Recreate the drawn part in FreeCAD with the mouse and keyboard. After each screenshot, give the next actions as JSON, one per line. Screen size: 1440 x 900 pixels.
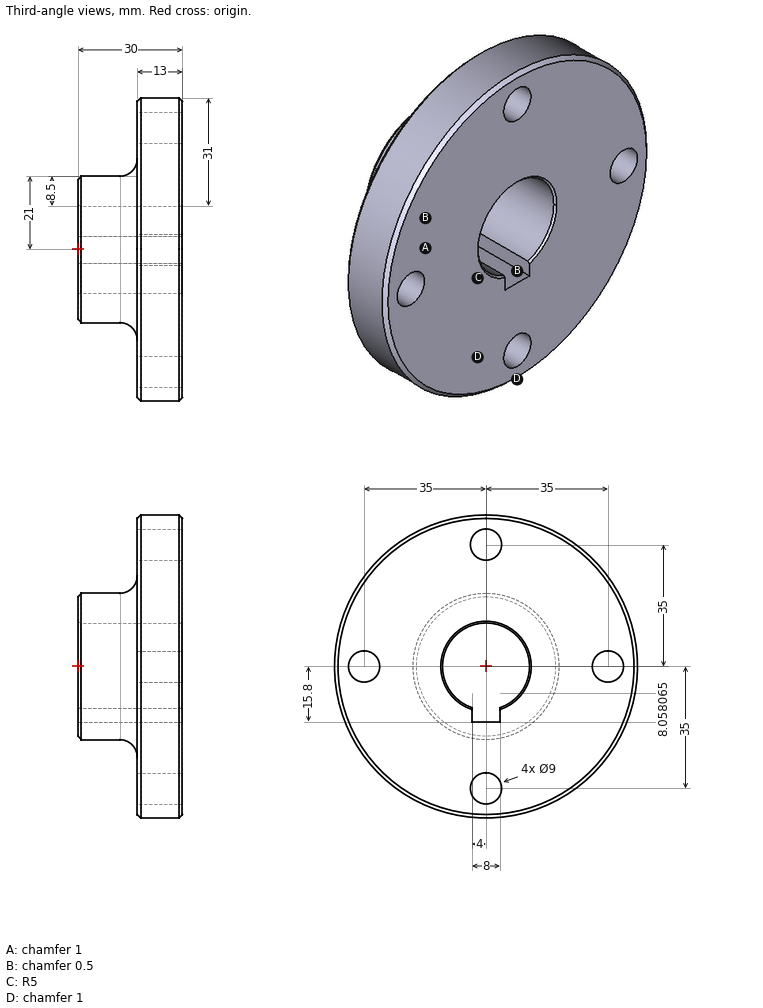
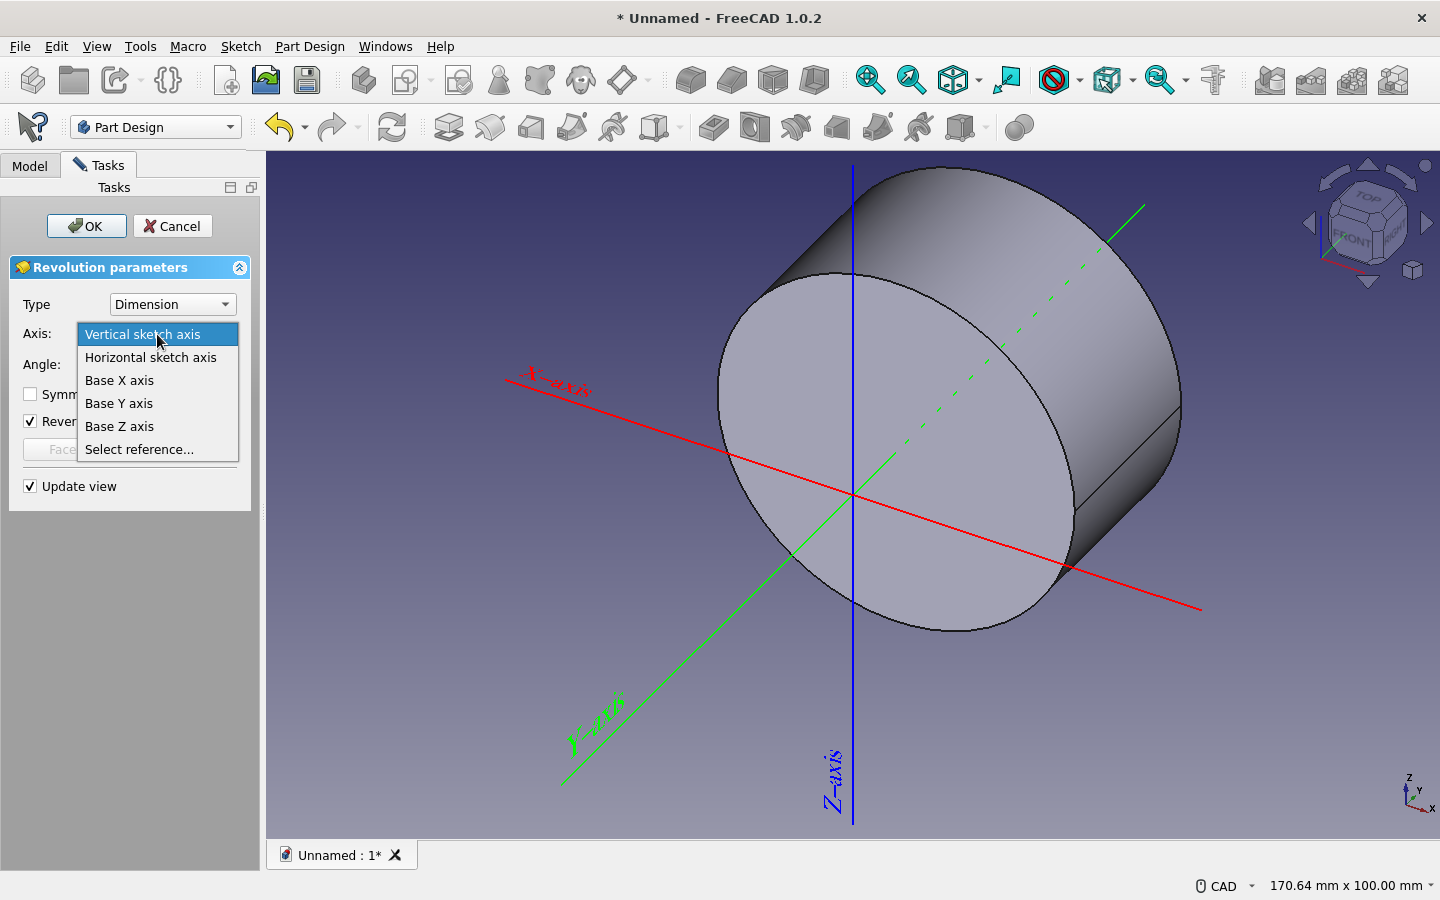
{"action": "left_click", "coordinate": [156, 358]}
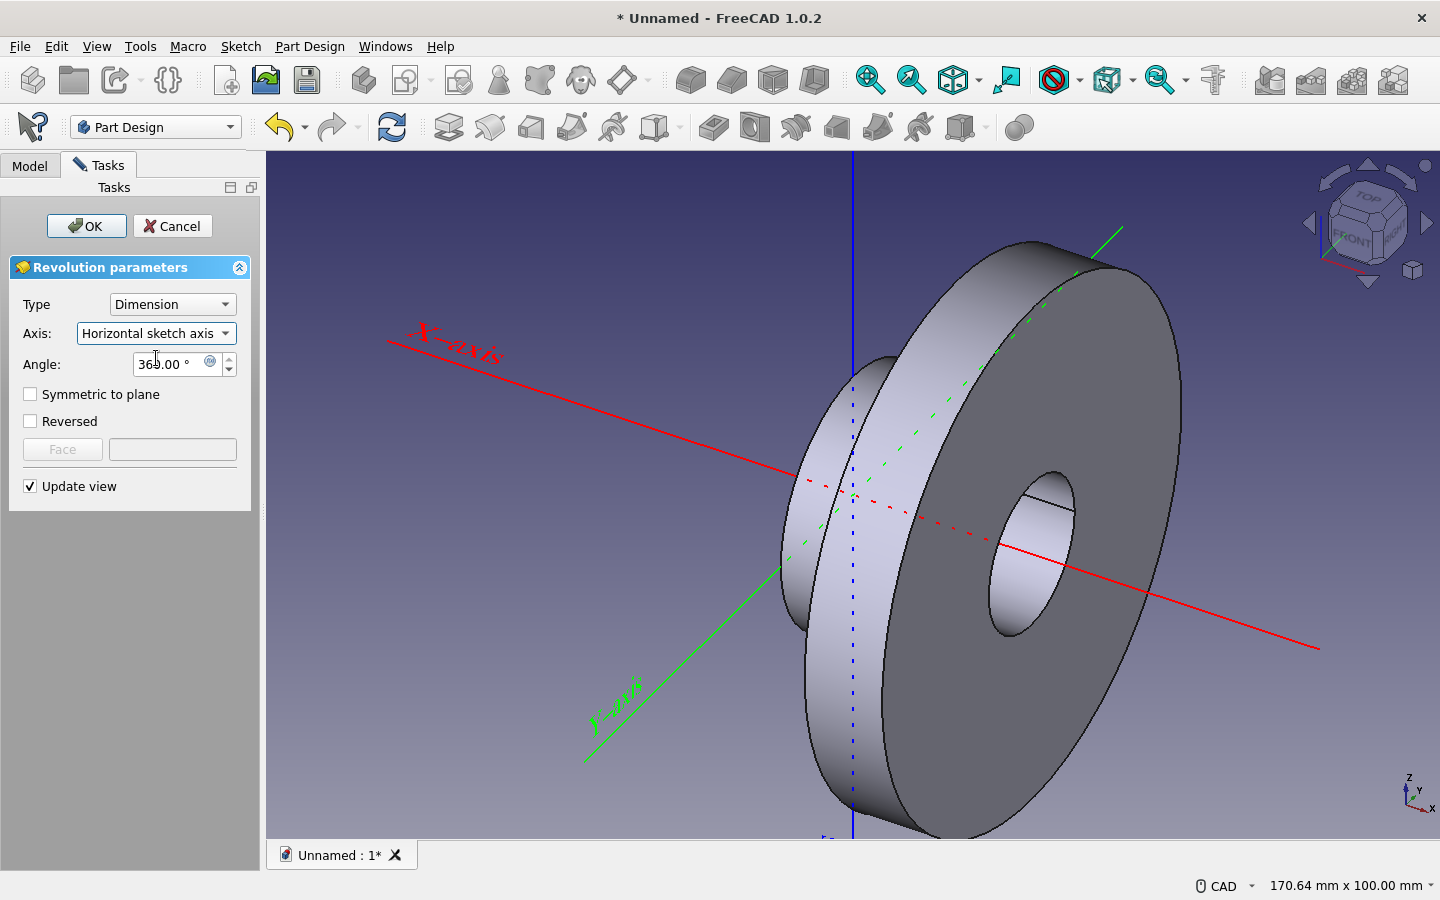
{"action": "left_click", "coordinate": [87, 226]}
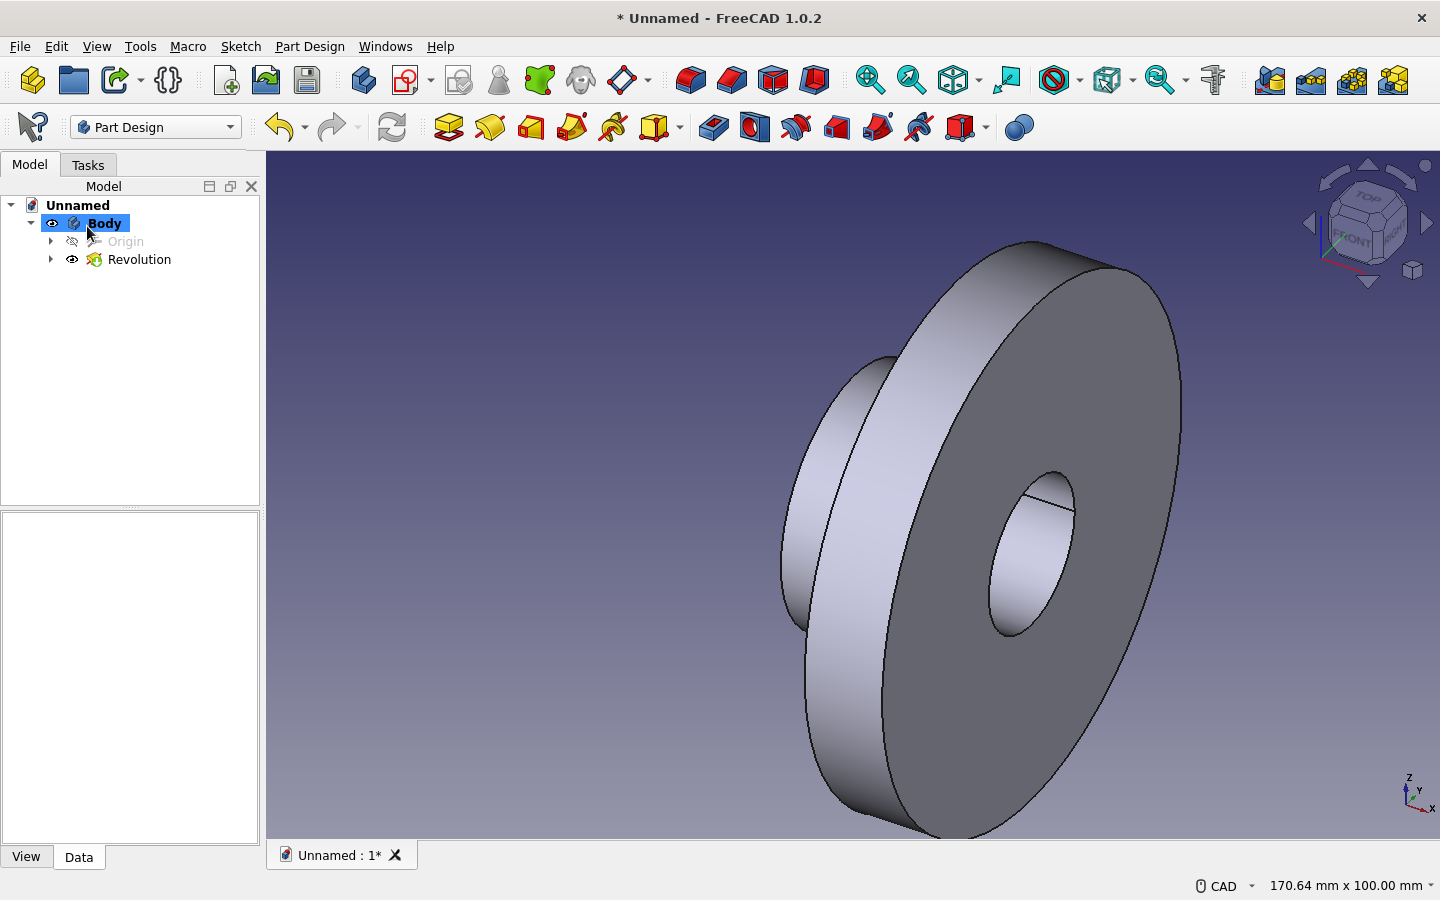
{"action": "left_click", "coordinate": [871, 80]}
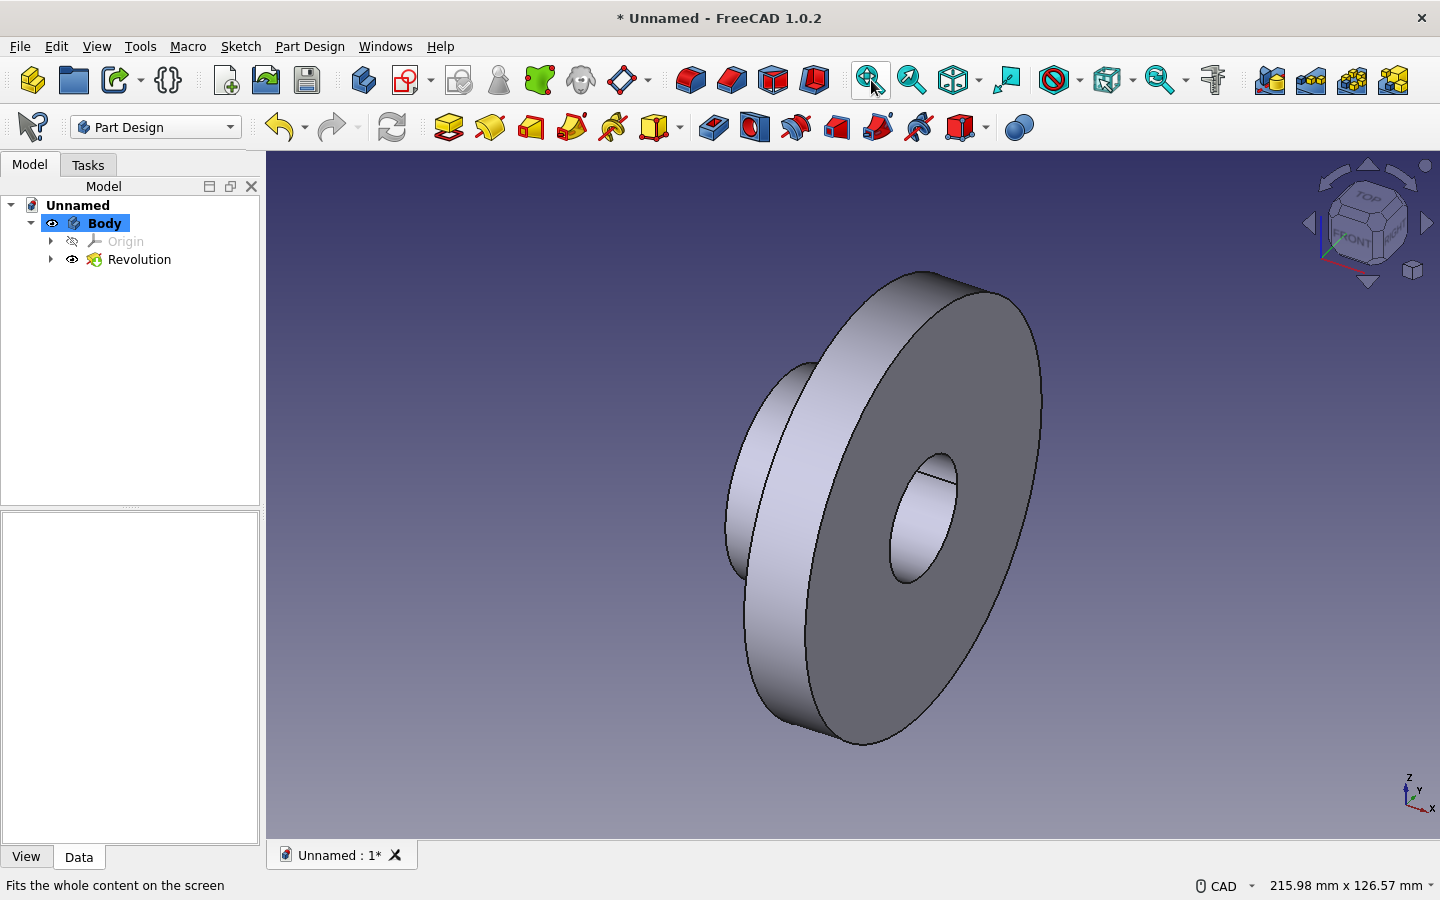
{"action": "key", "text": "0"}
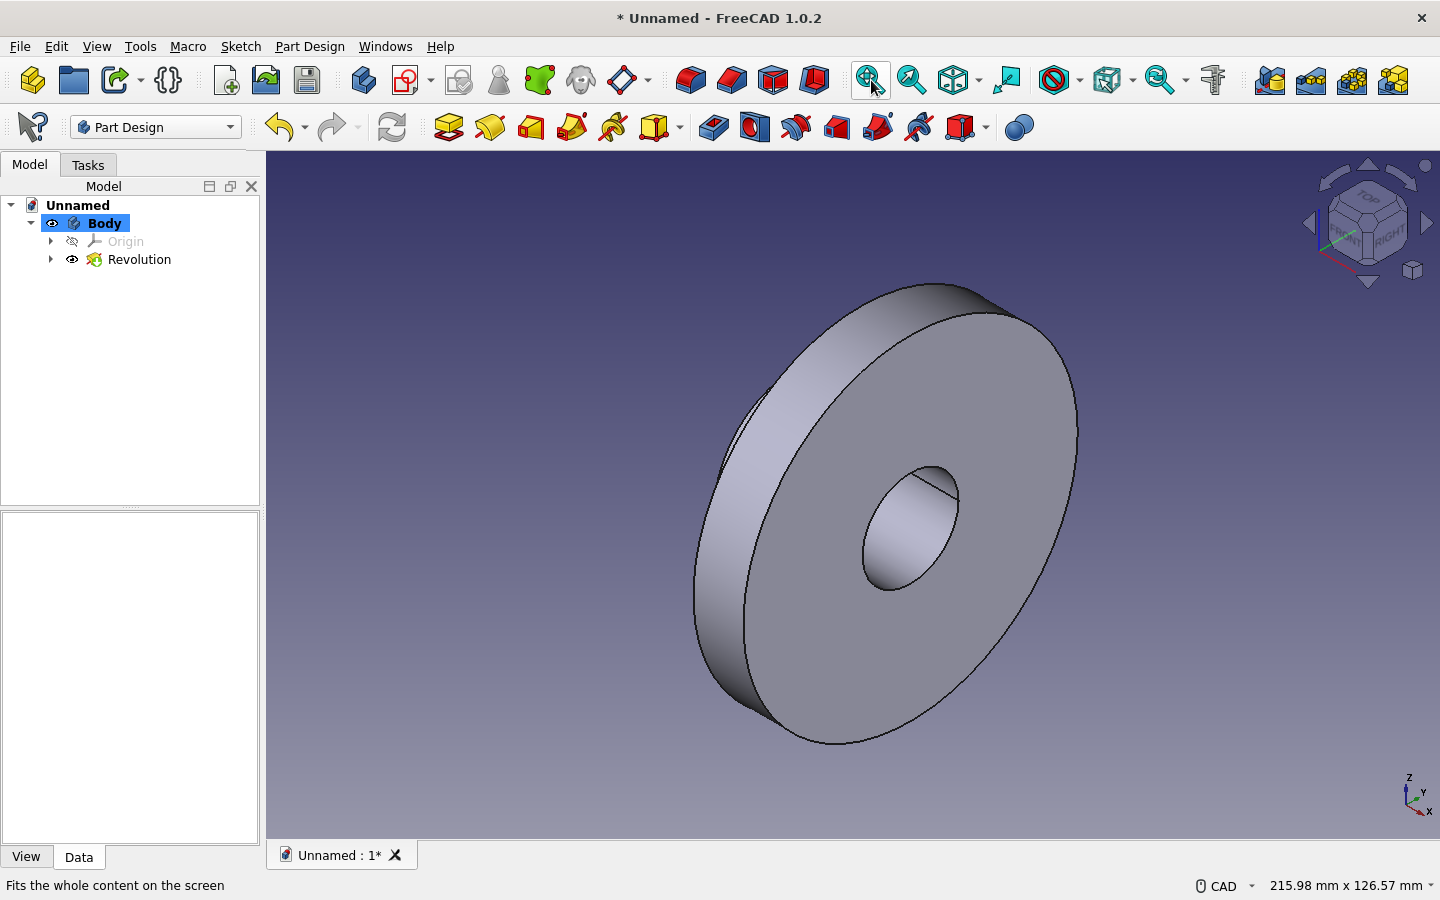
{"action": "key", "text": "2"}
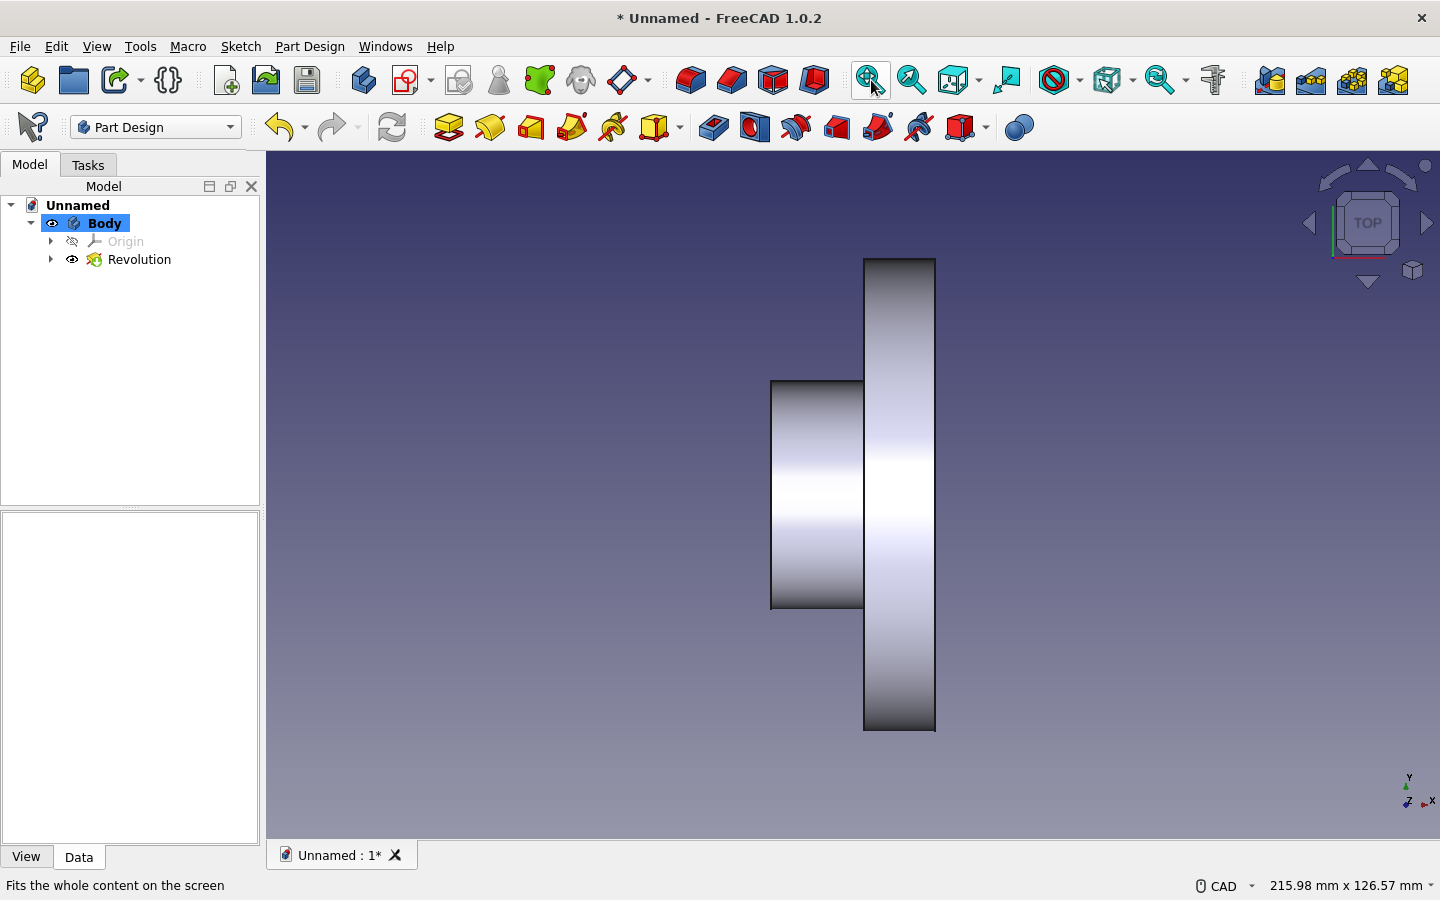
{"action": "left_click", "coordinate": [771, 587]}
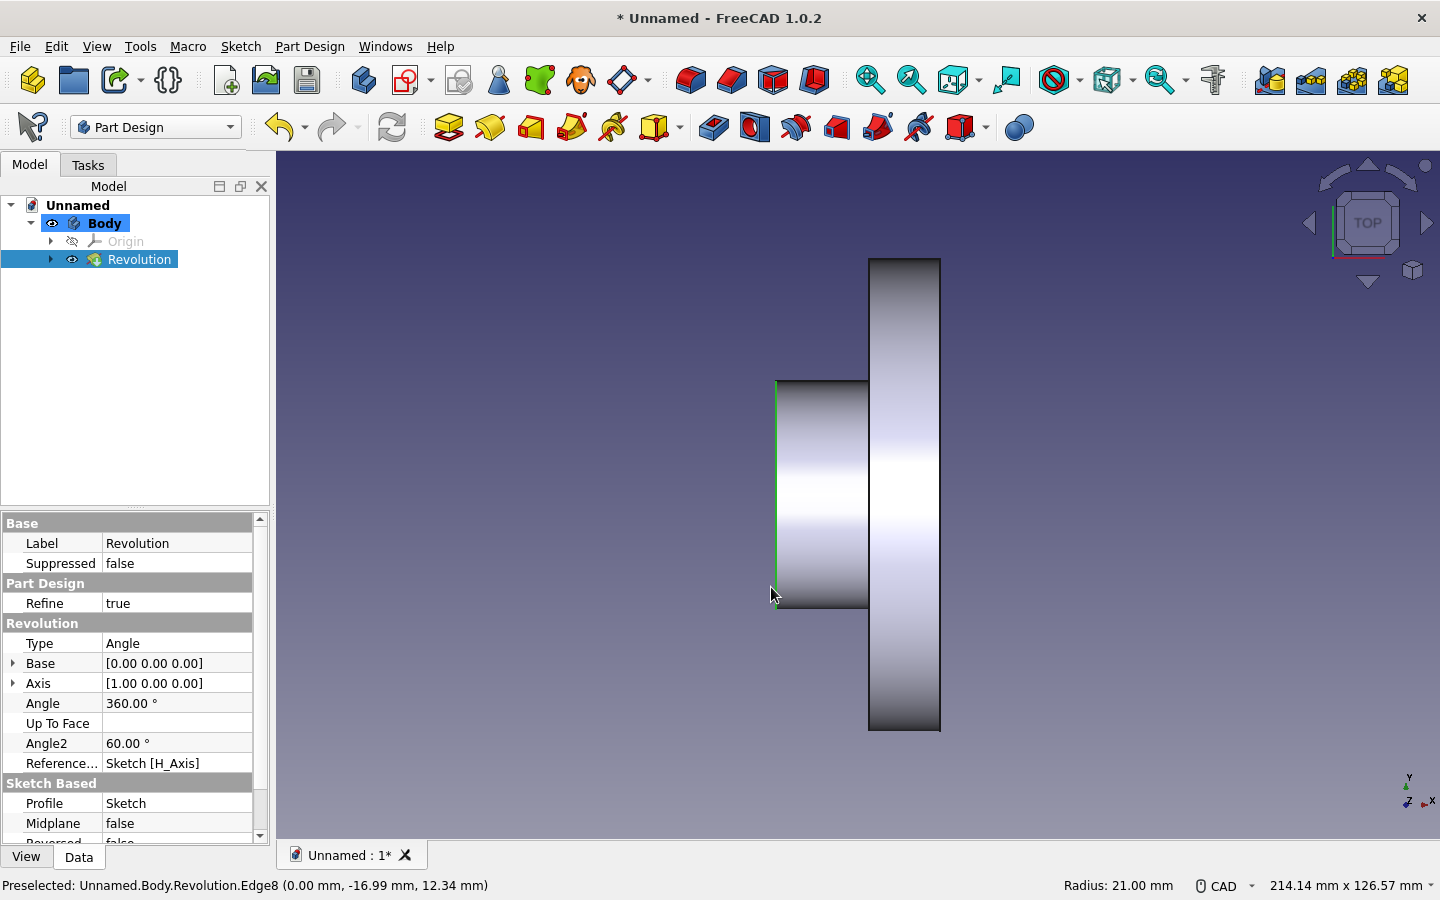
{"action": "left_click", "coordinate": [732, 80]}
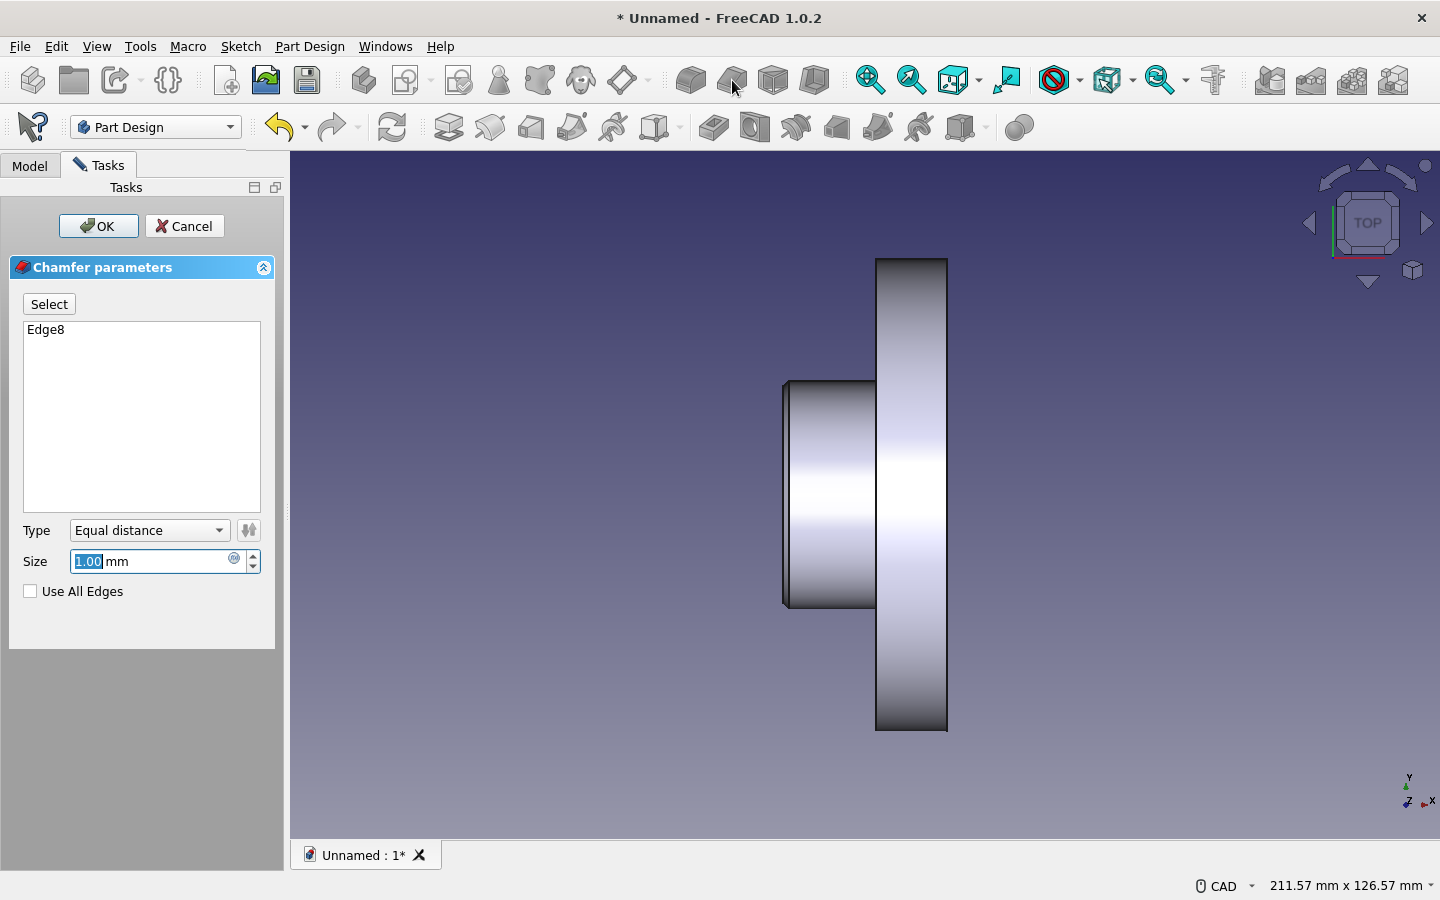
{"action": "type", "text": "1"}
{"action": "key", "text": "Tab"}